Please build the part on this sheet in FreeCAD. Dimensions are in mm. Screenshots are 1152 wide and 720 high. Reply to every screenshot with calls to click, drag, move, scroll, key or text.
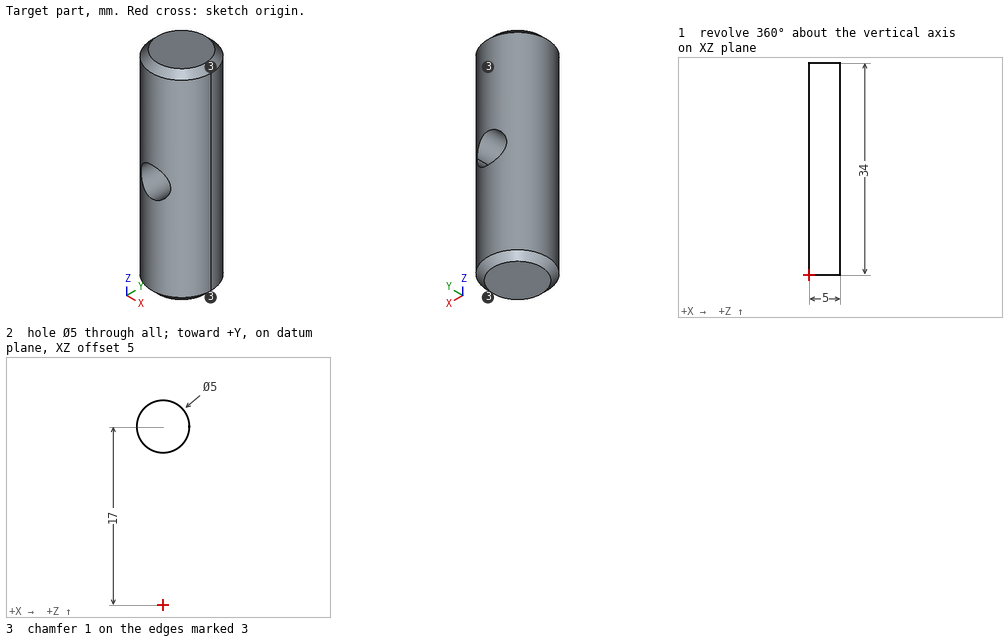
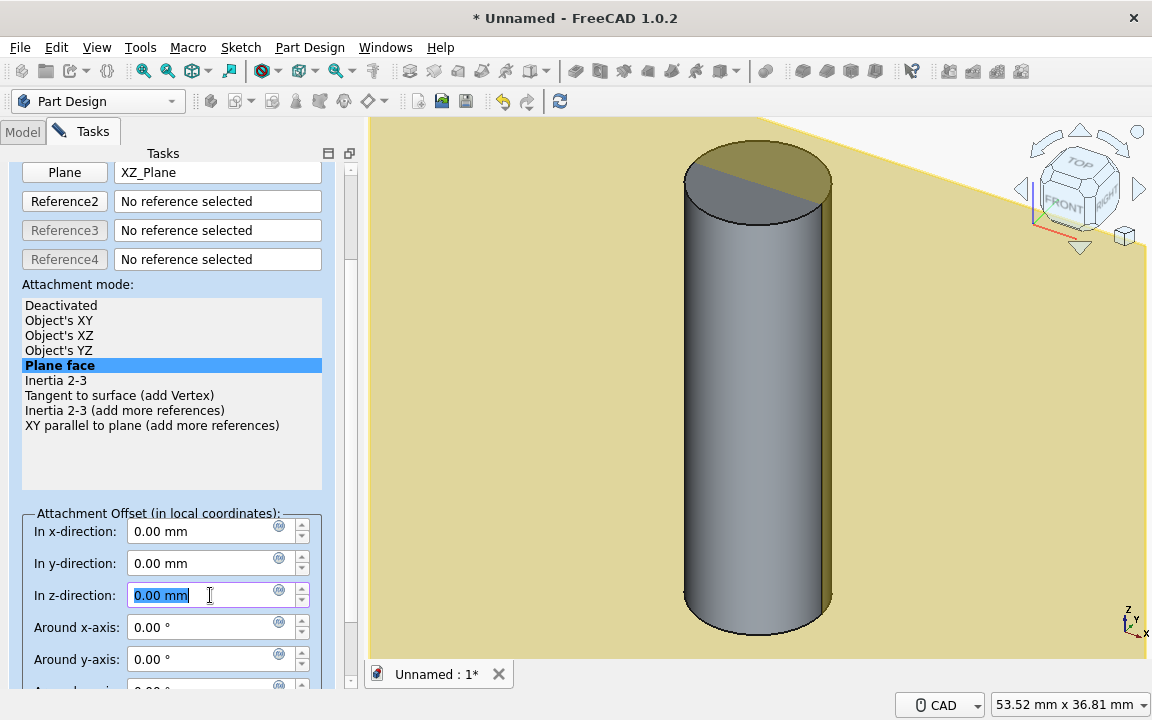
text(5)
key(Tab)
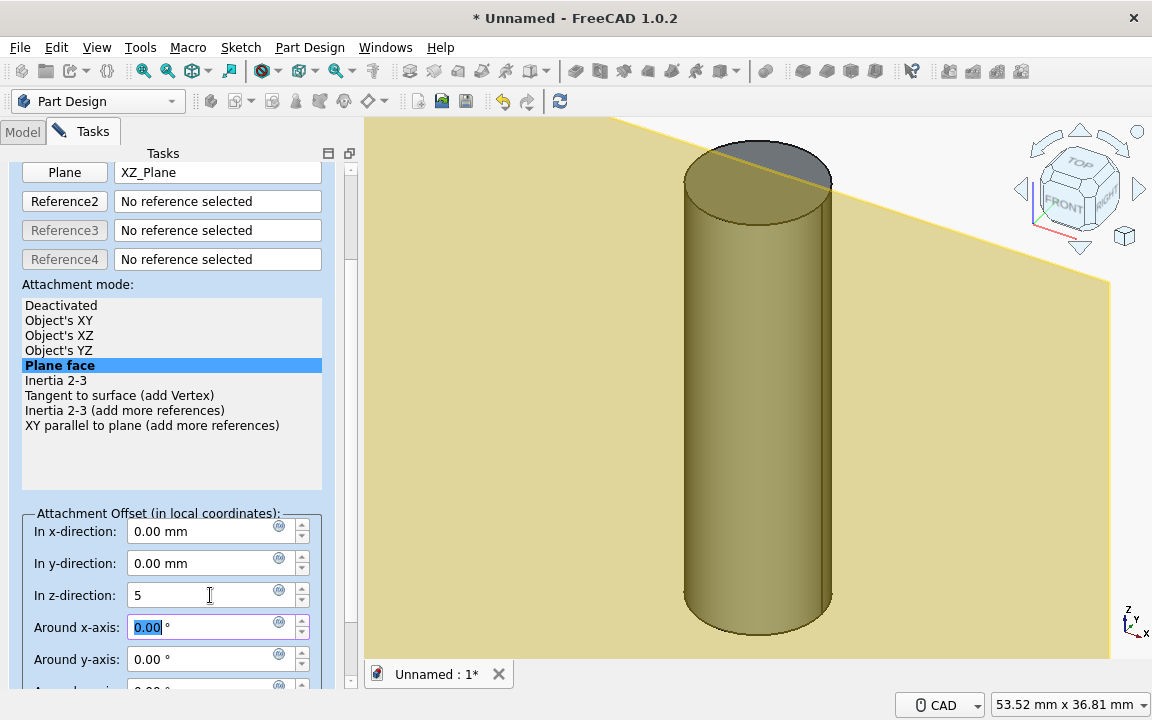
scroll(351, 426, up, 3)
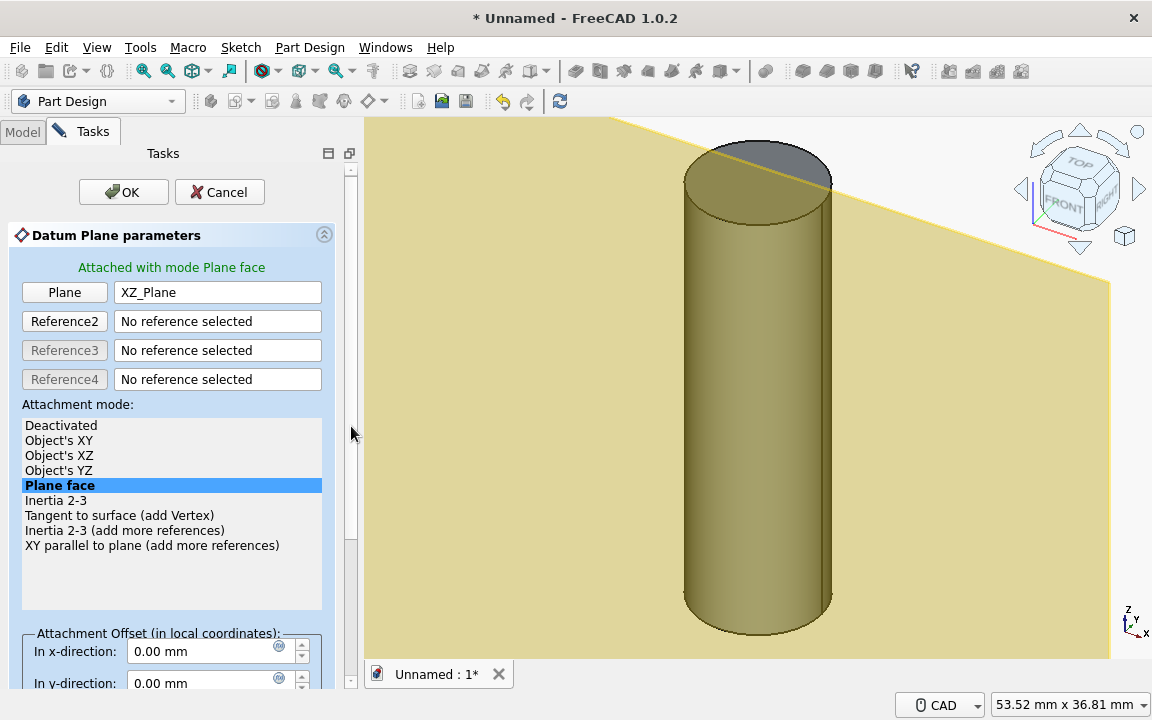
click(124, 192)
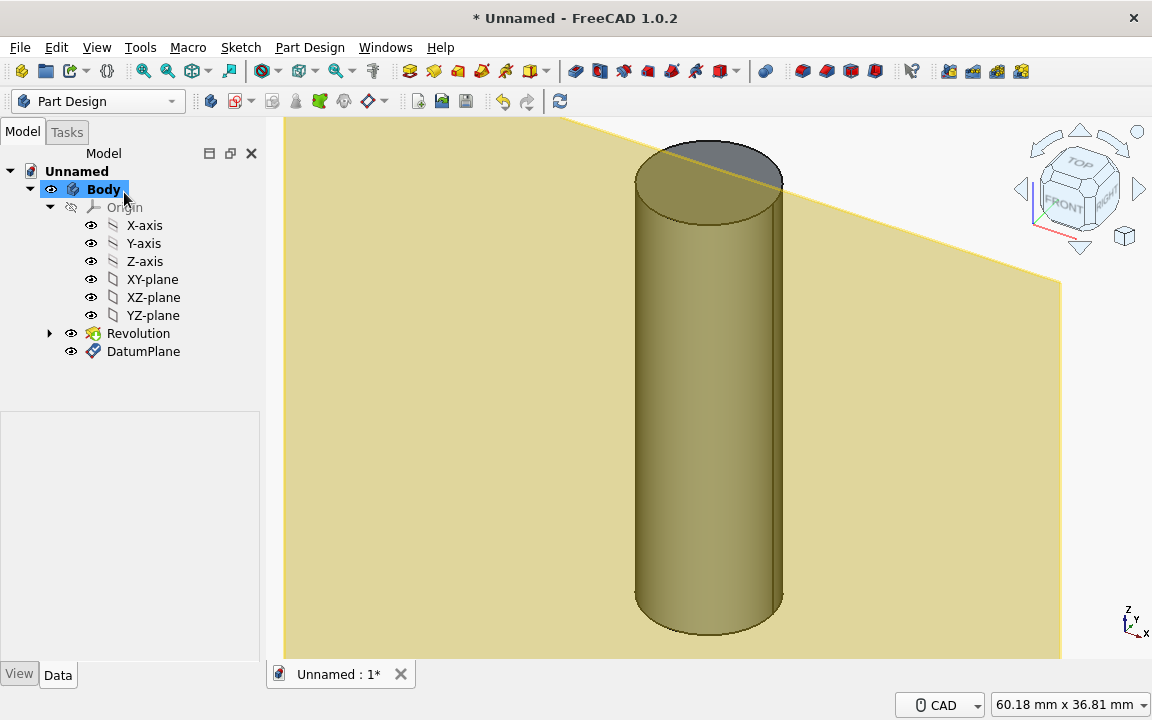
click(116, 351)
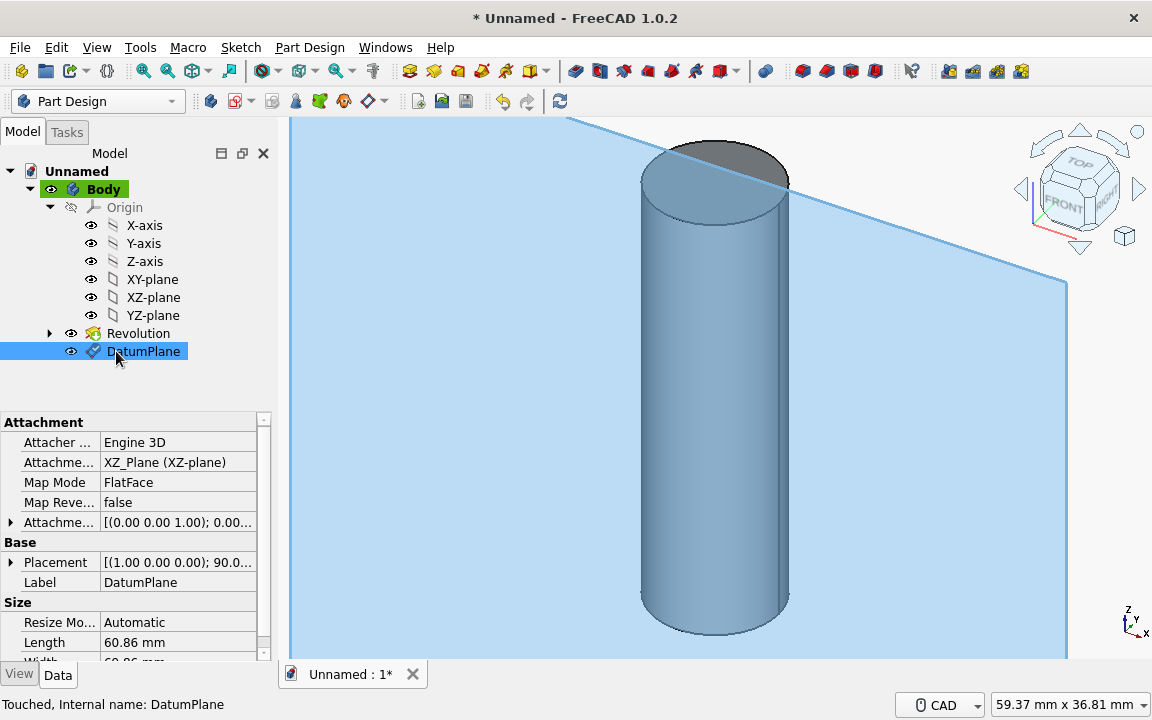
click(236, 102)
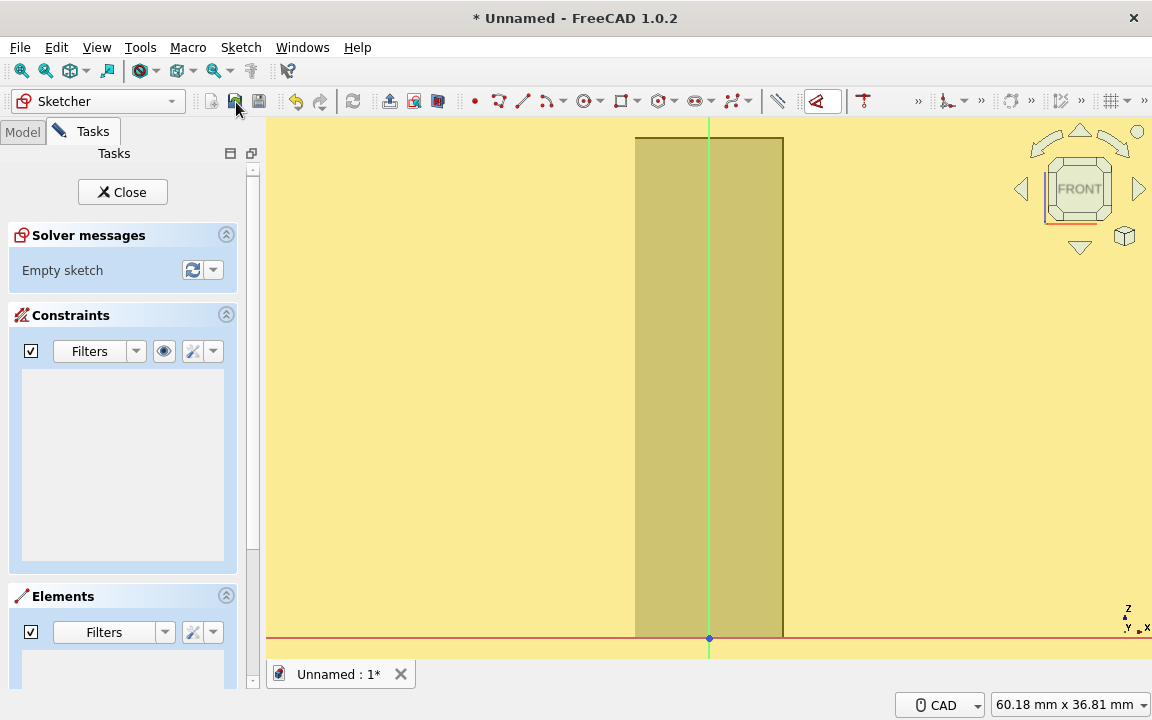
scroll(726, 388, up, 8)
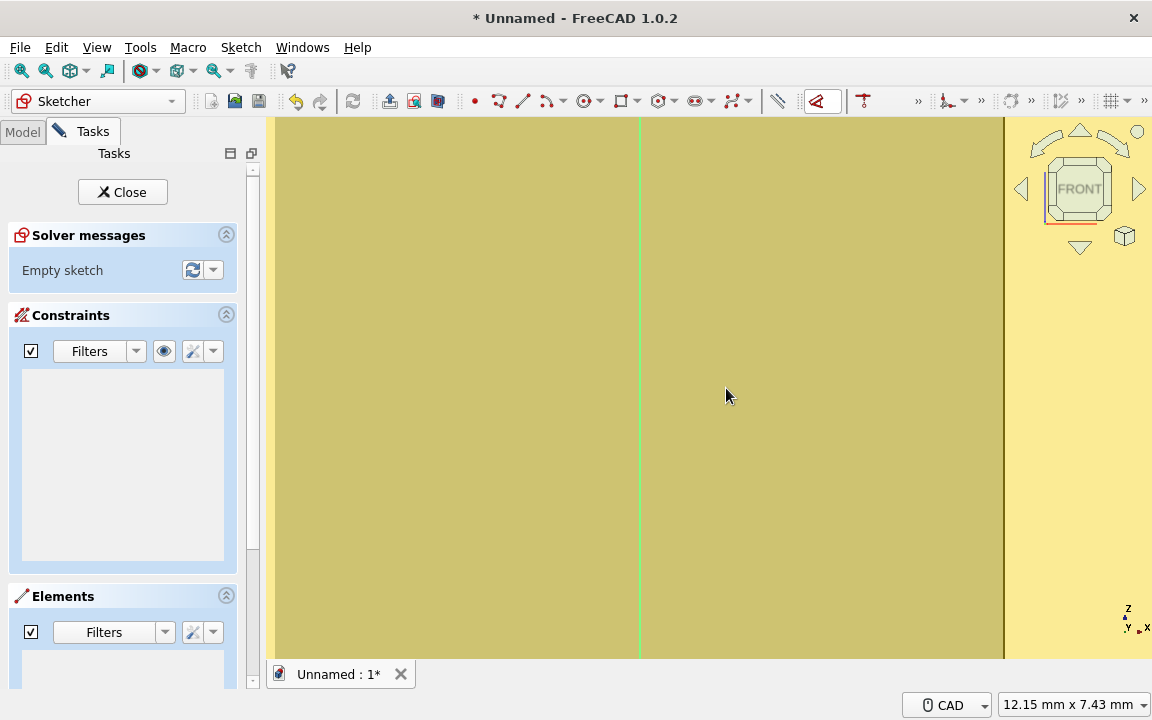
click(584, 102)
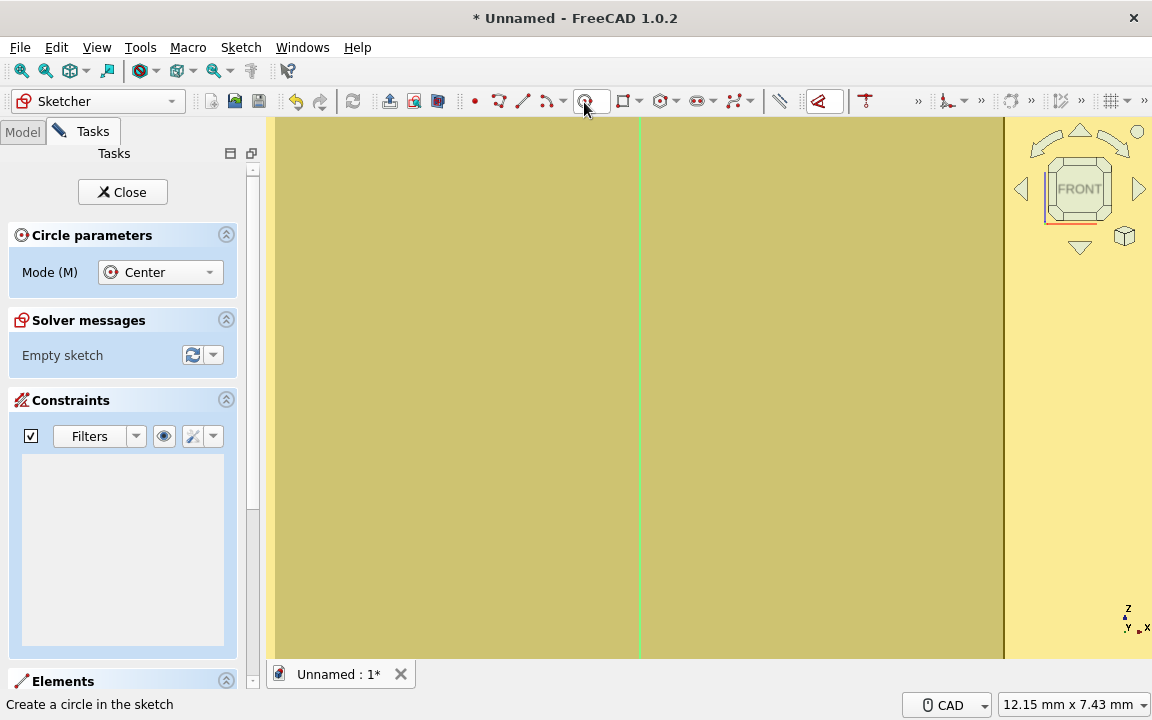
click(640, 386)
click(769, 257)
key(Escape)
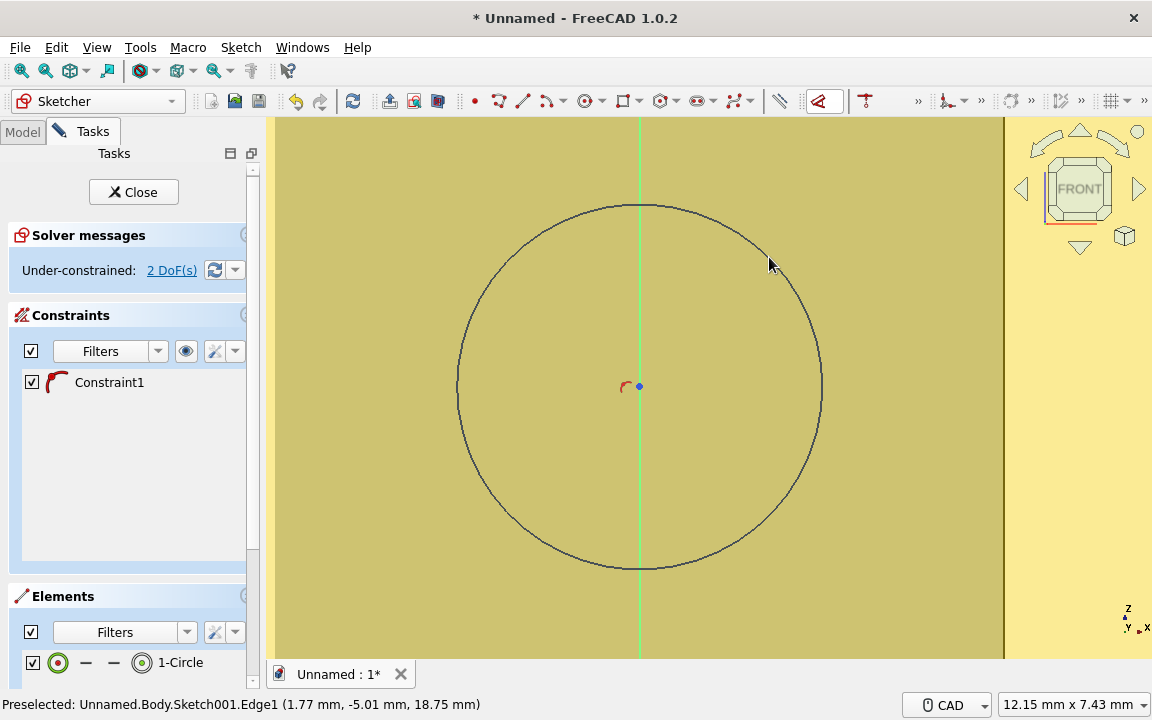
click(768, 257)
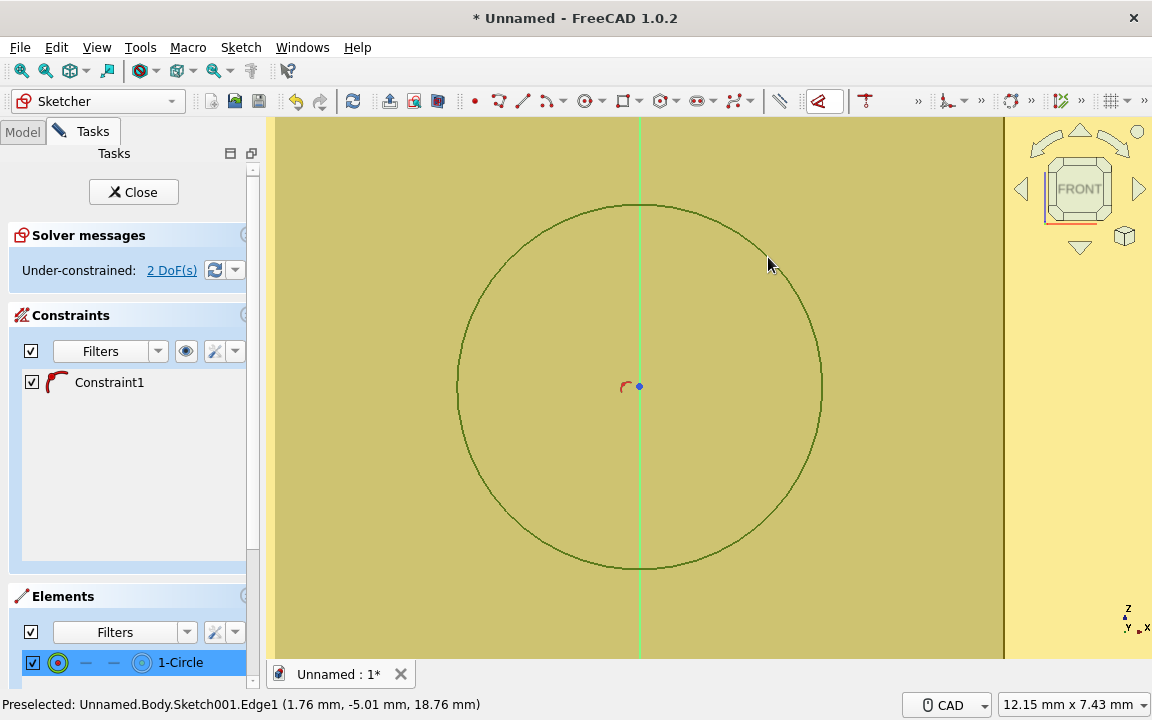
click(838, 102)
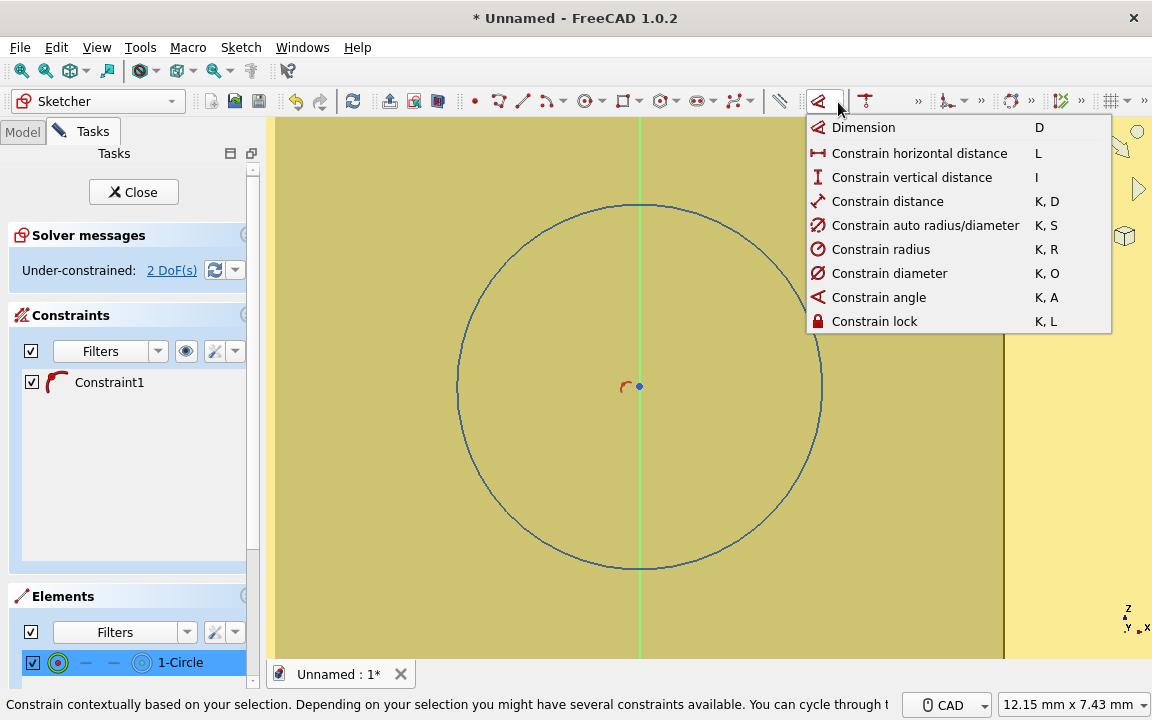
click(959, 273)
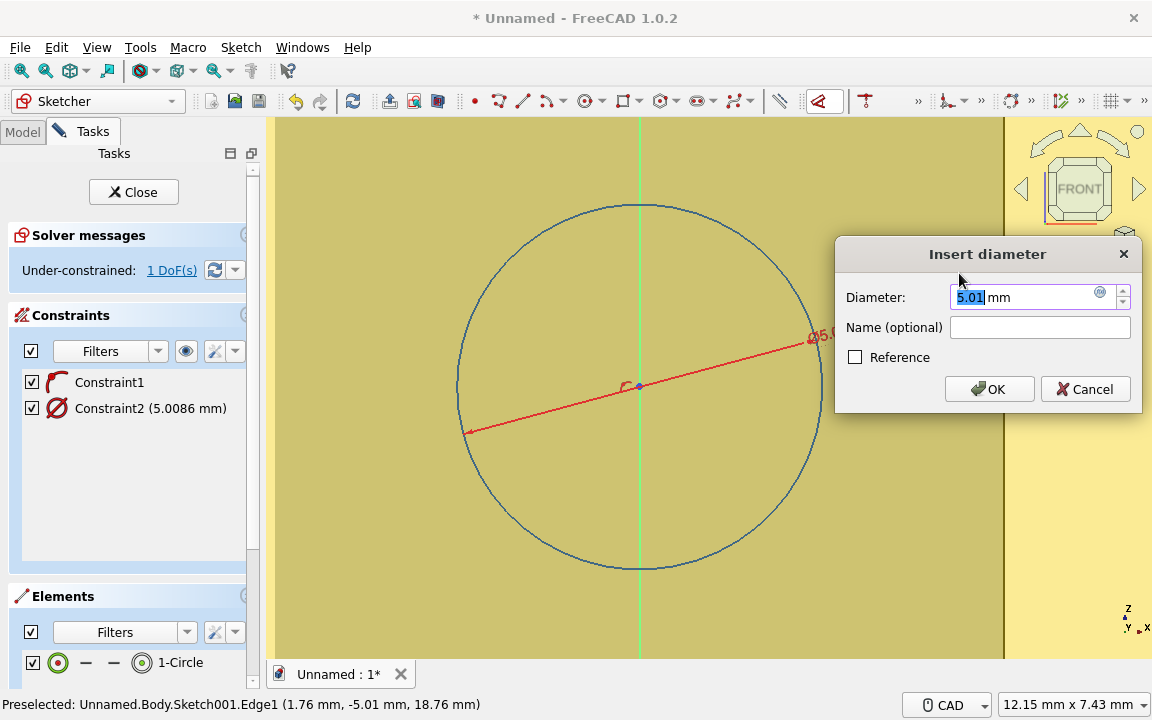
text(5)
key(Return)